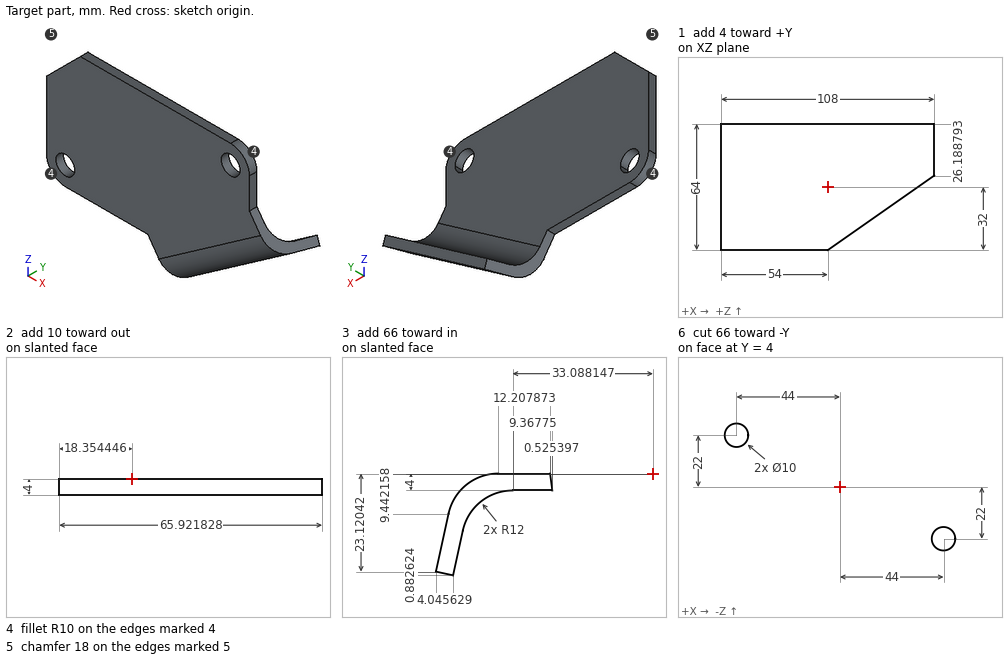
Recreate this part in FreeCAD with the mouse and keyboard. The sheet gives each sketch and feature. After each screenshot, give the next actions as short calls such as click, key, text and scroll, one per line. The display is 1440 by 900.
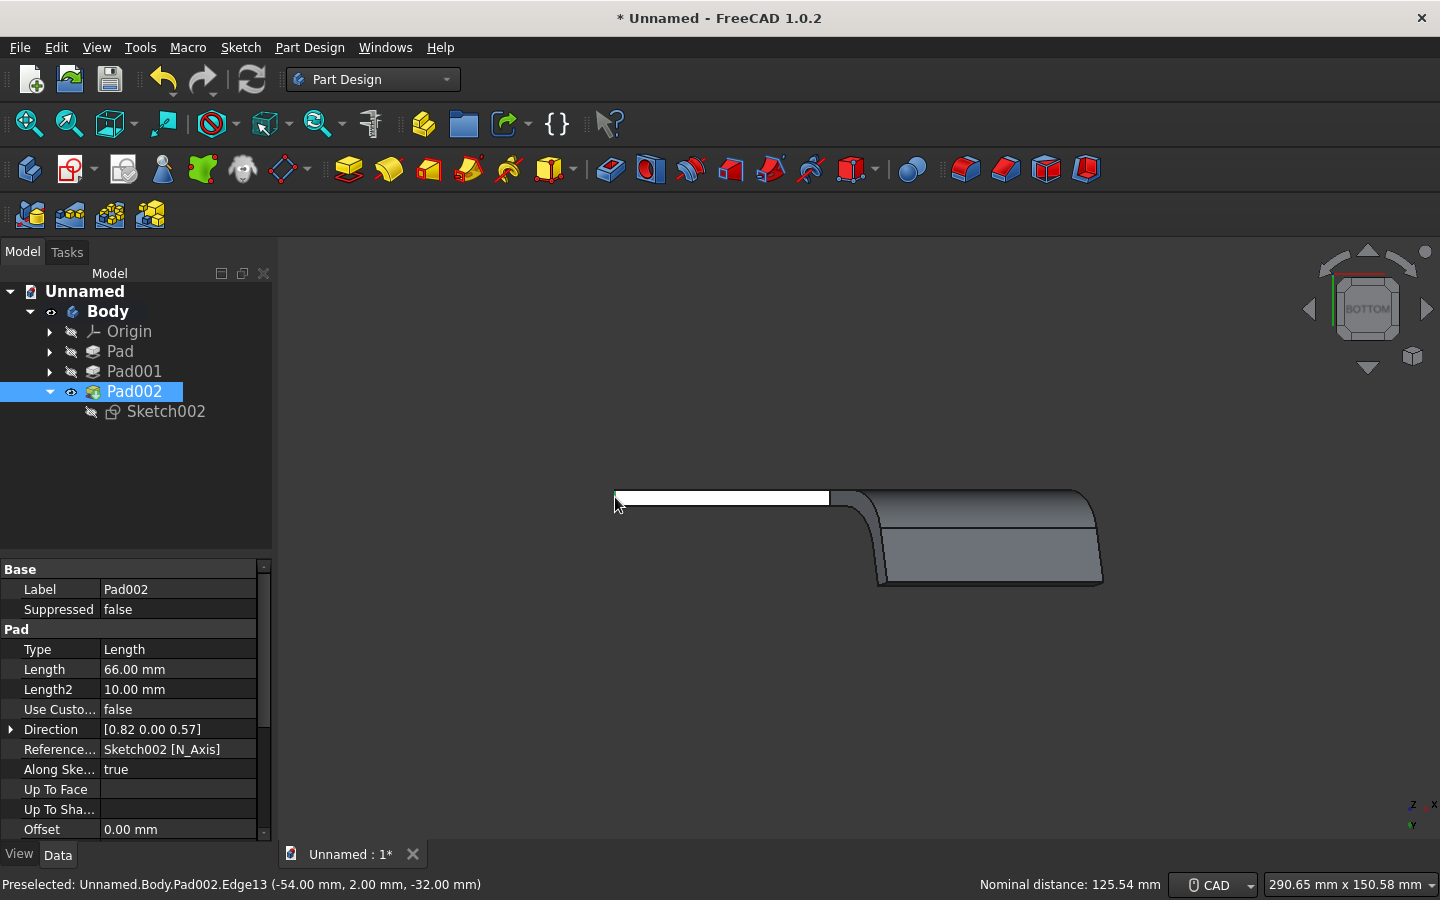
click(966, 170)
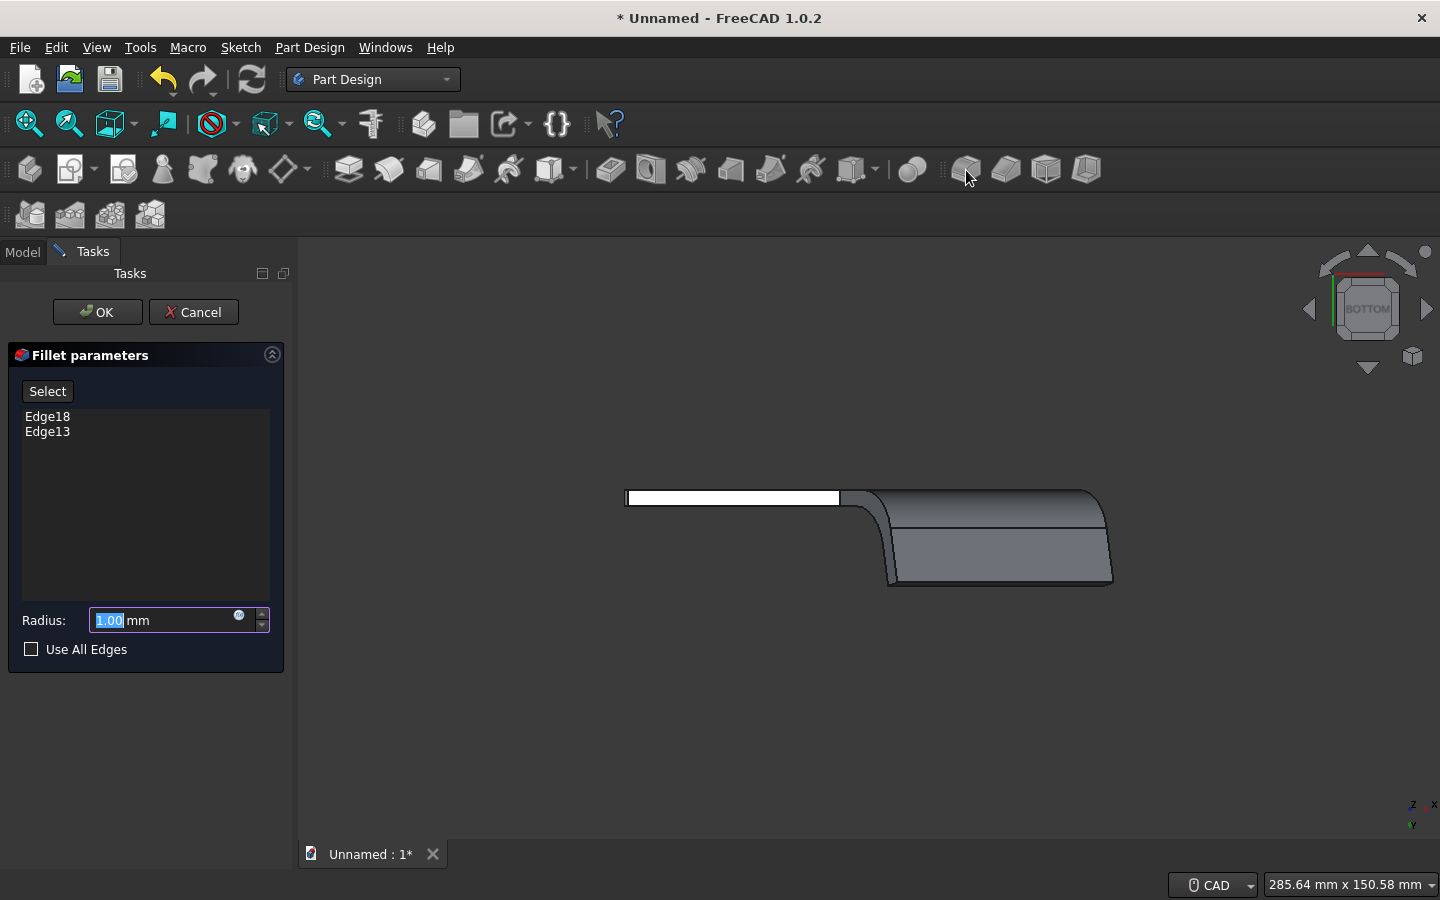
text(10)
key(Tab)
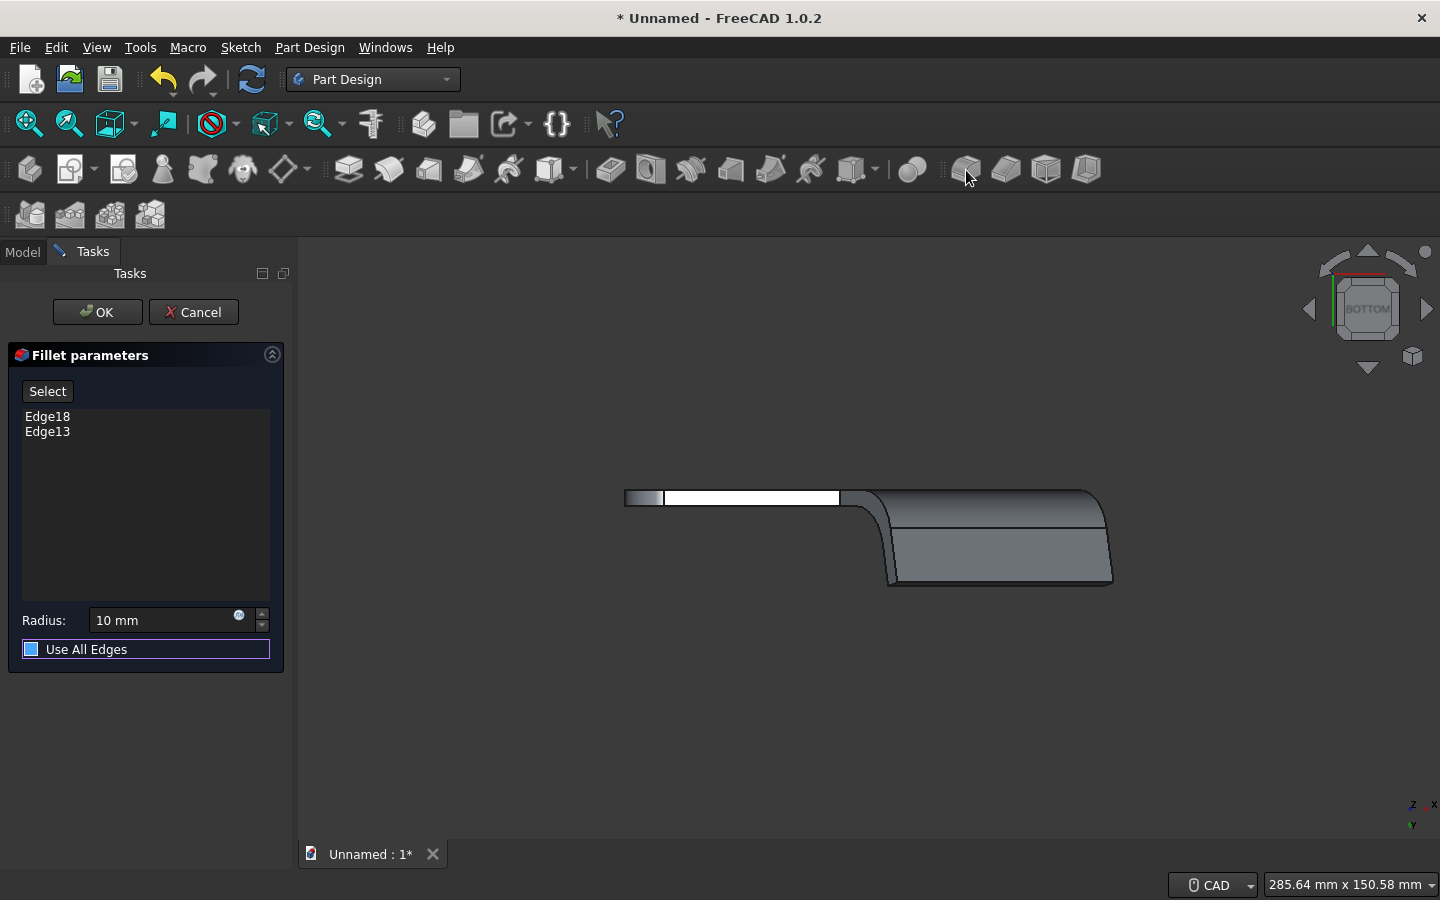
click(98, 312)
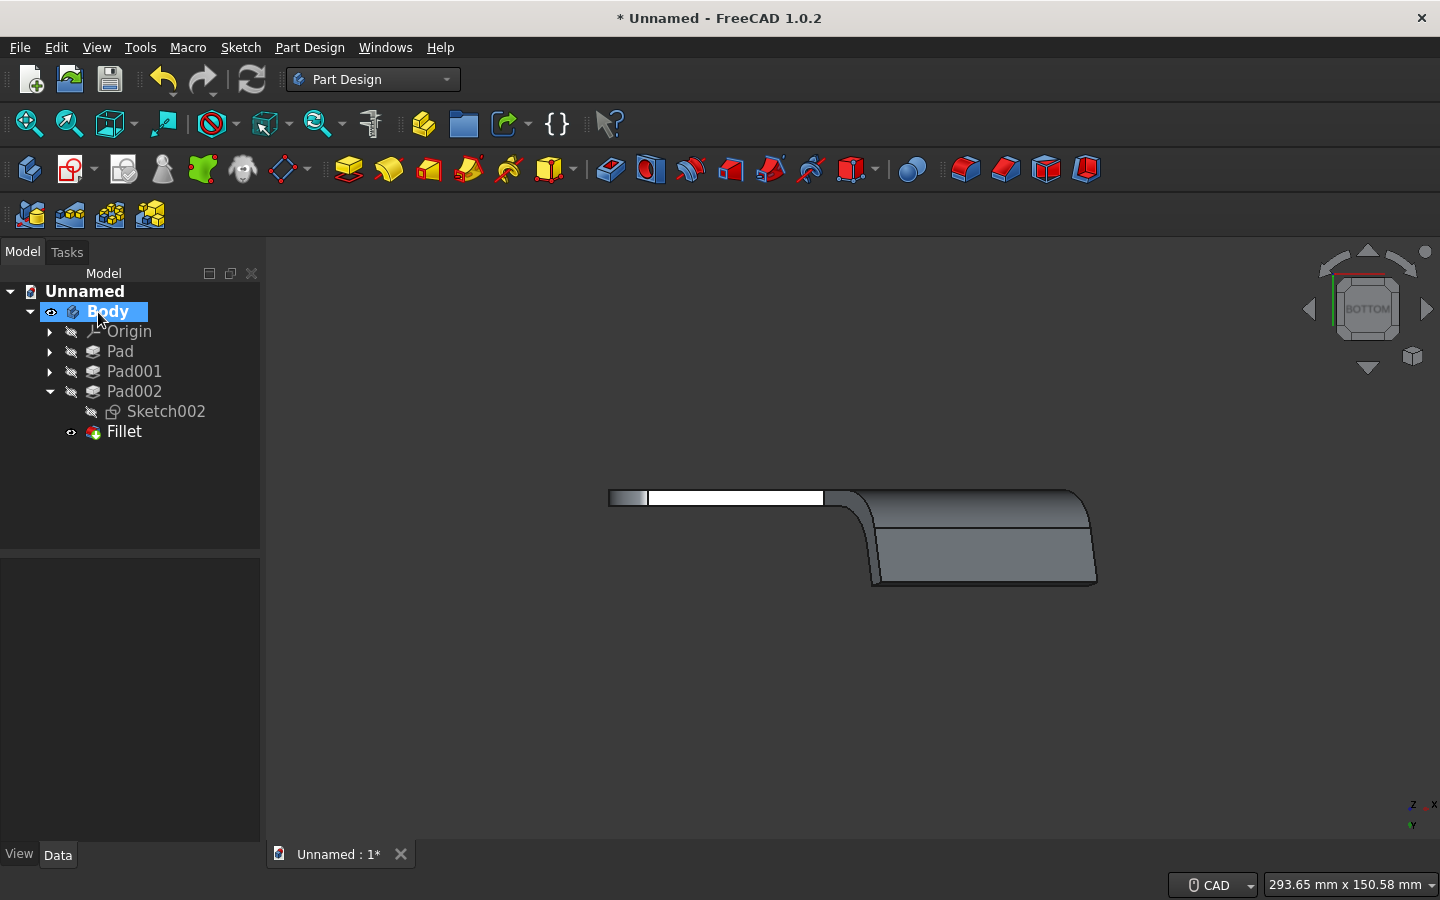
click(30, 124)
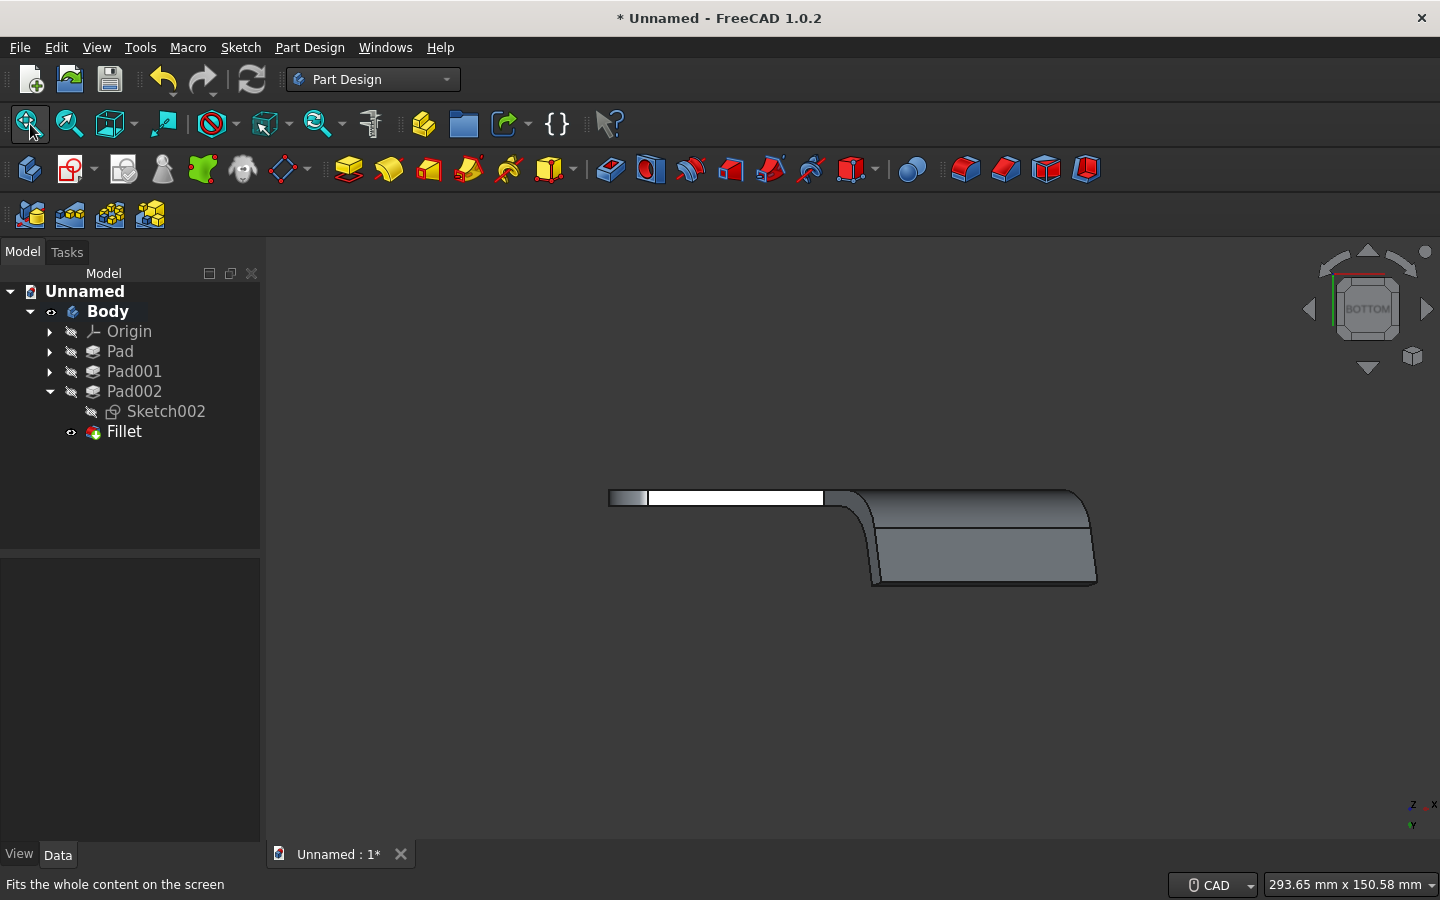
scroll(609, 497, up, 5)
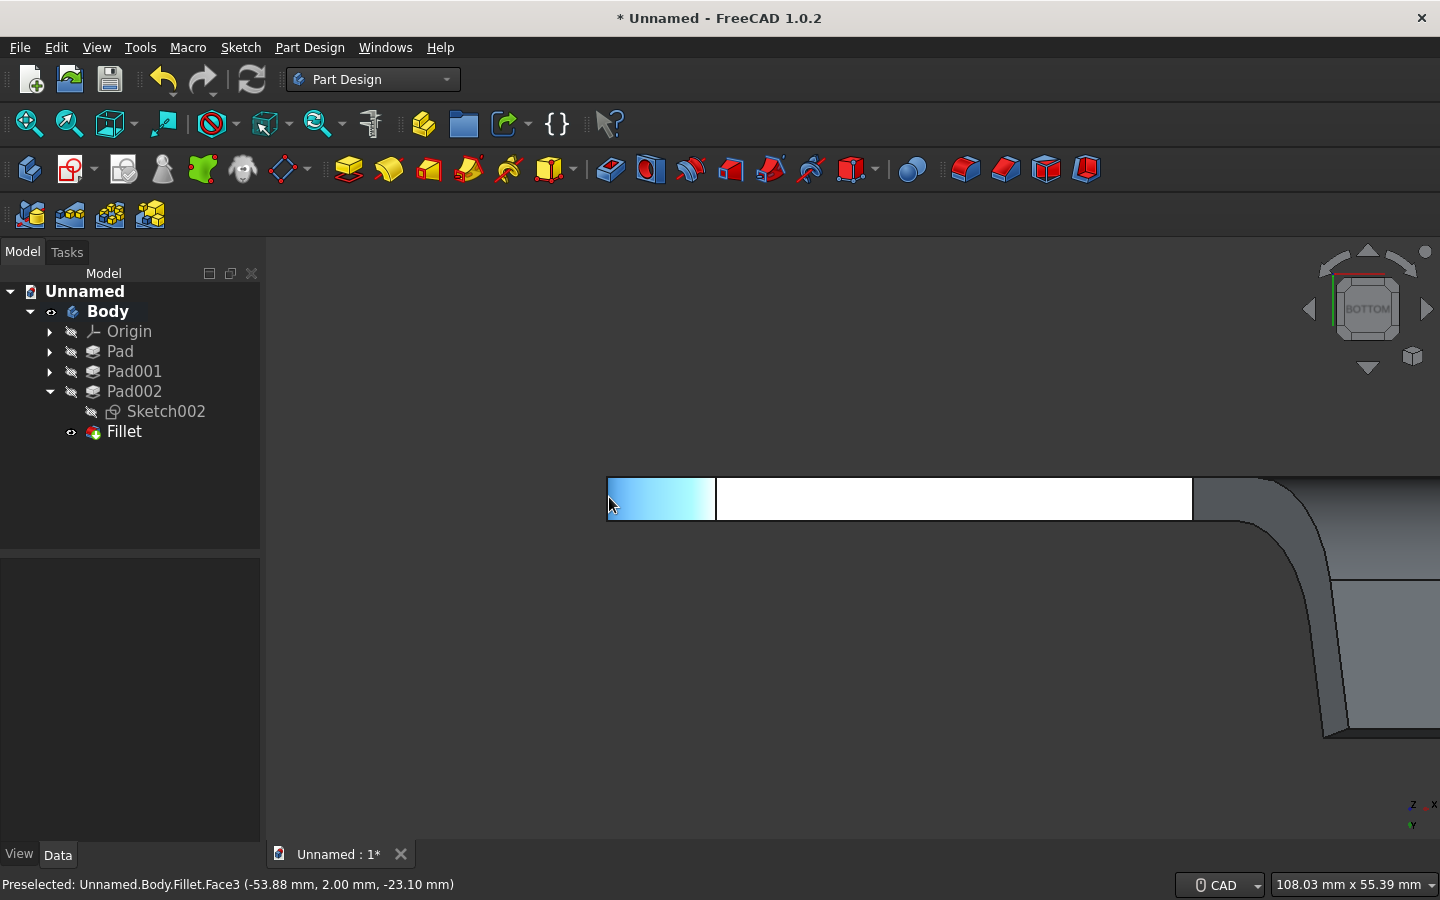
key(v)
key(f)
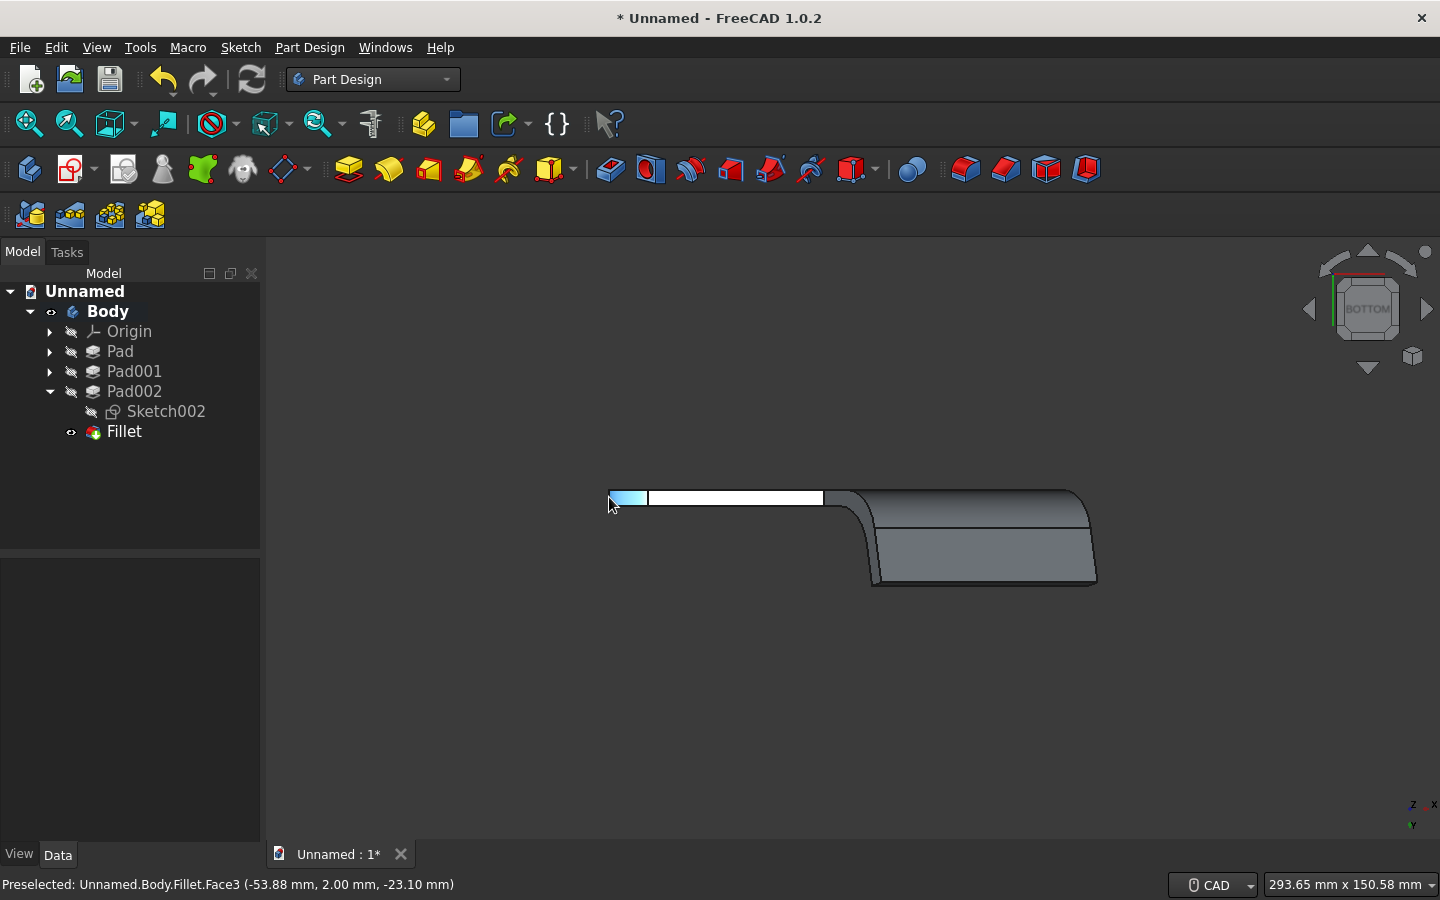
key(0)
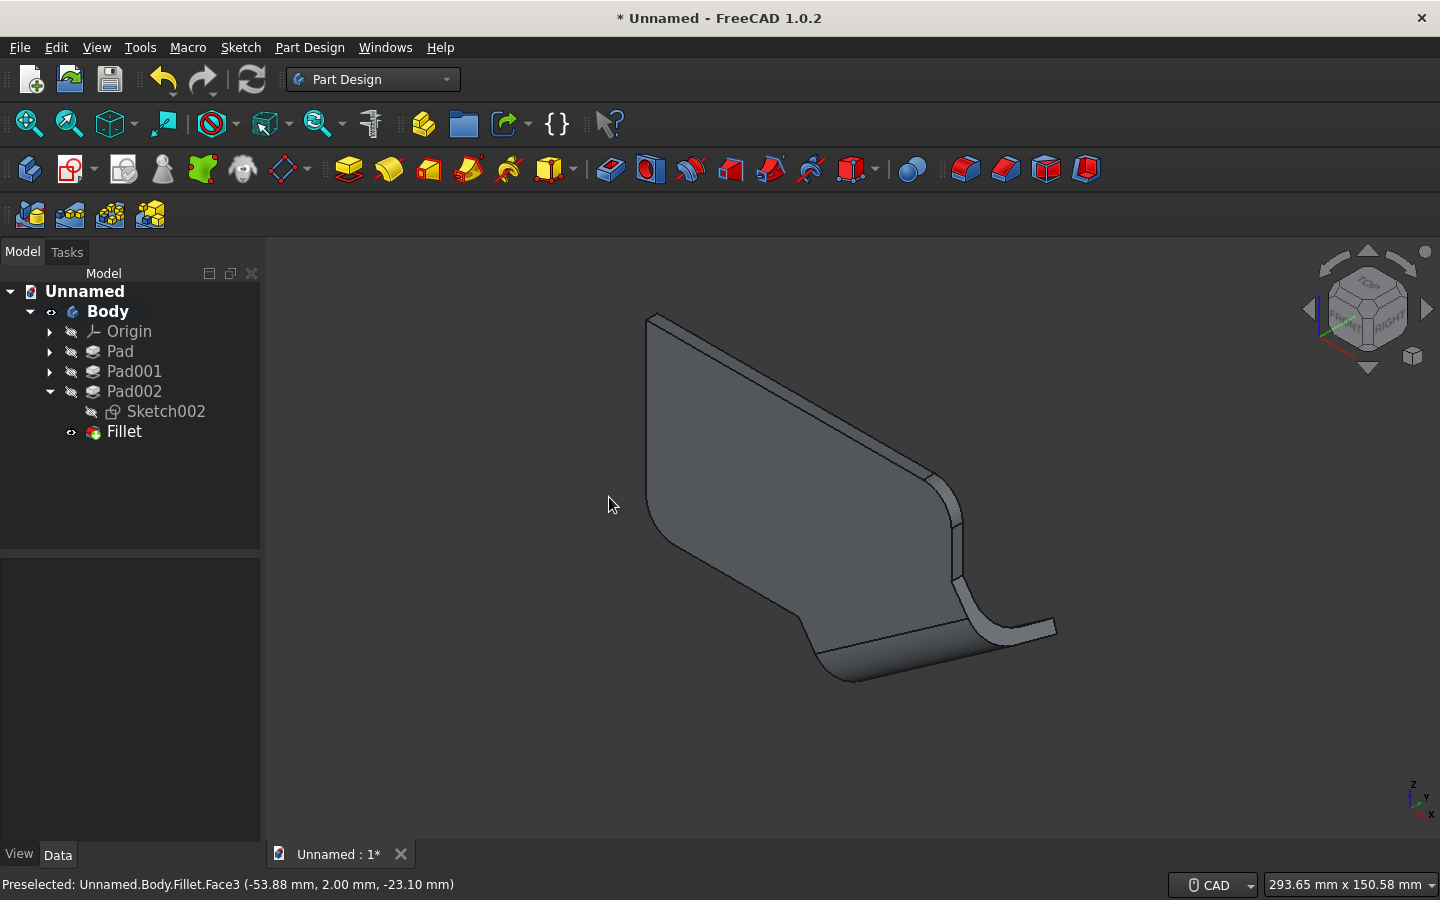
scroll(652, 316, up, 5)